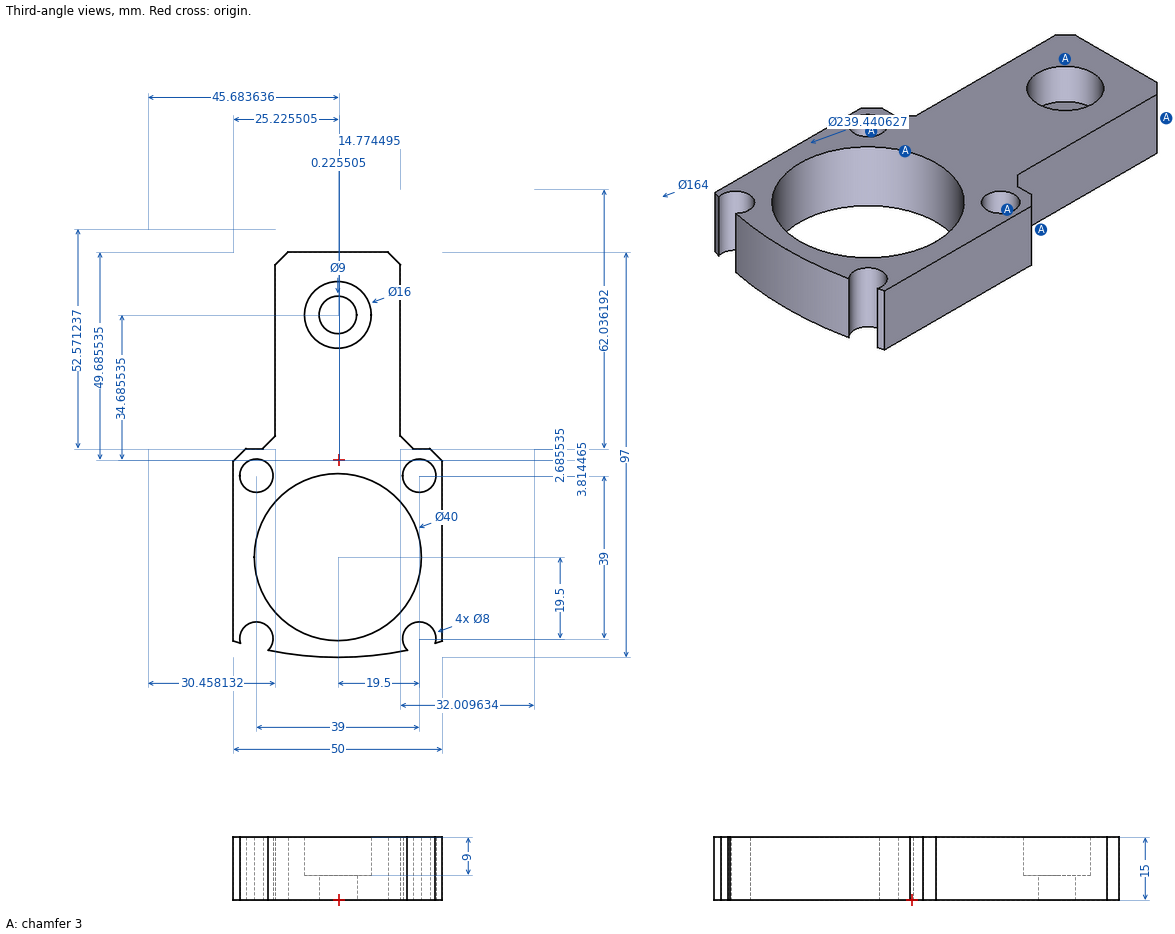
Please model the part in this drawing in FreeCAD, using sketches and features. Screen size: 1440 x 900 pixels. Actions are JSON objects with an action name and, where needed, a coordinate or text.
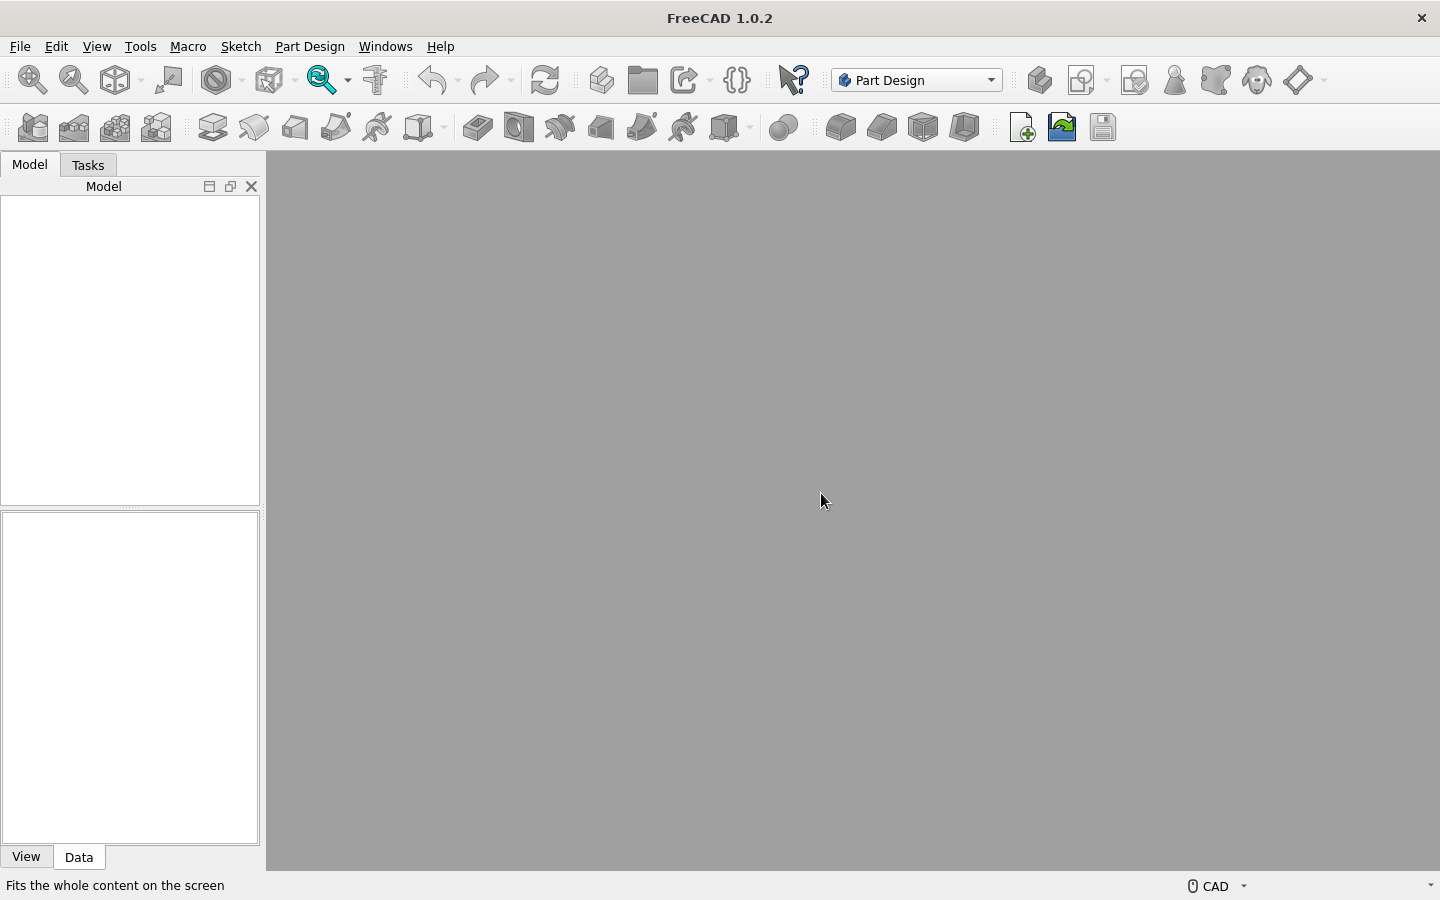
{"action": "left_click", "coordinate": [1021, 128]}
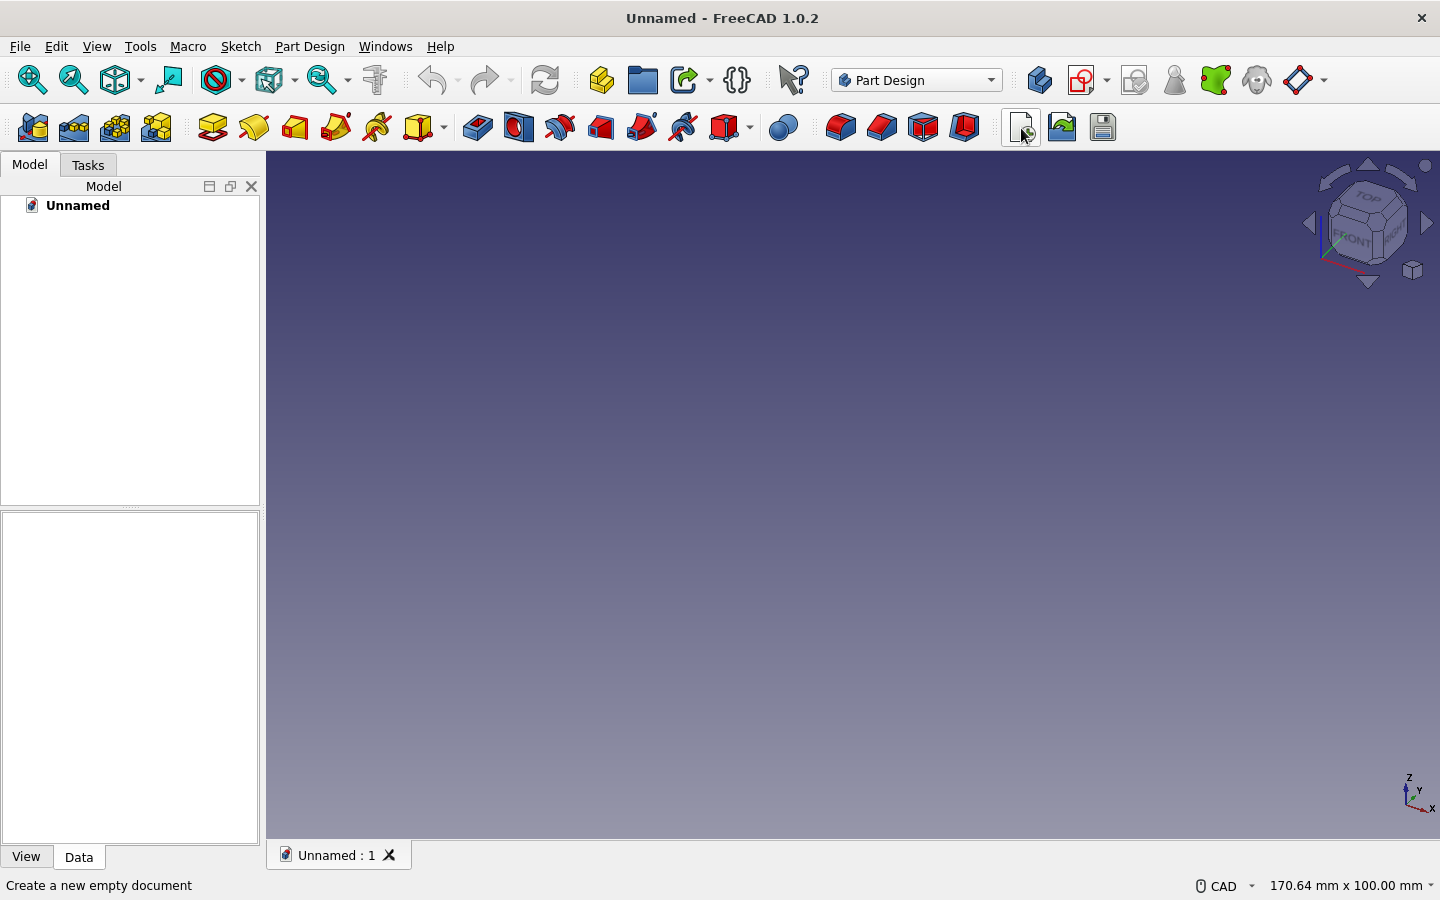
{"action": "left_click", "coordinate": [1080, 80]}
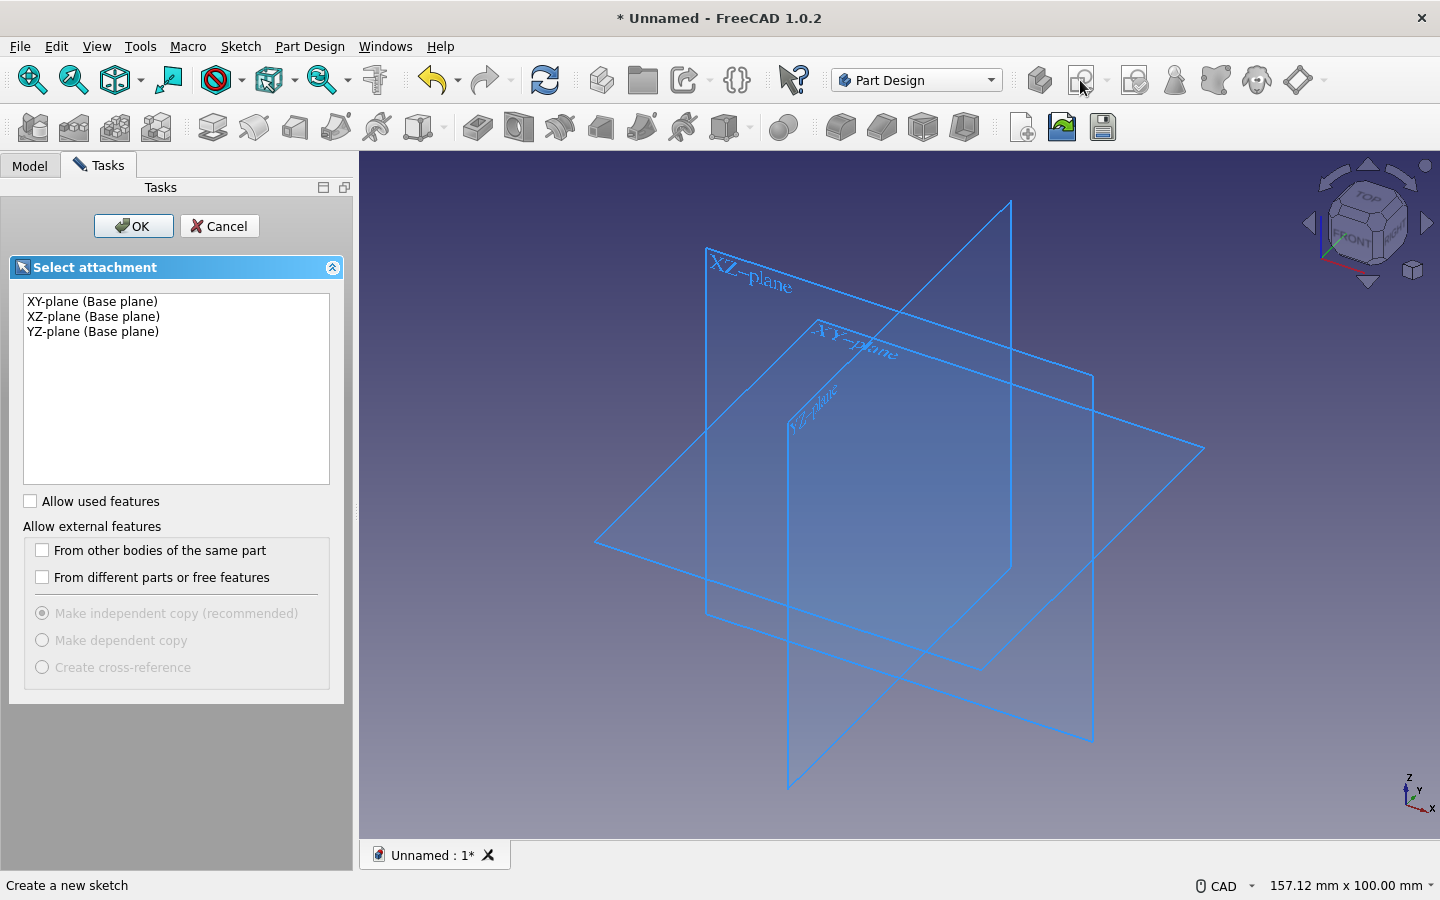
{"action": "left_click", "coordinate": [84, 302]}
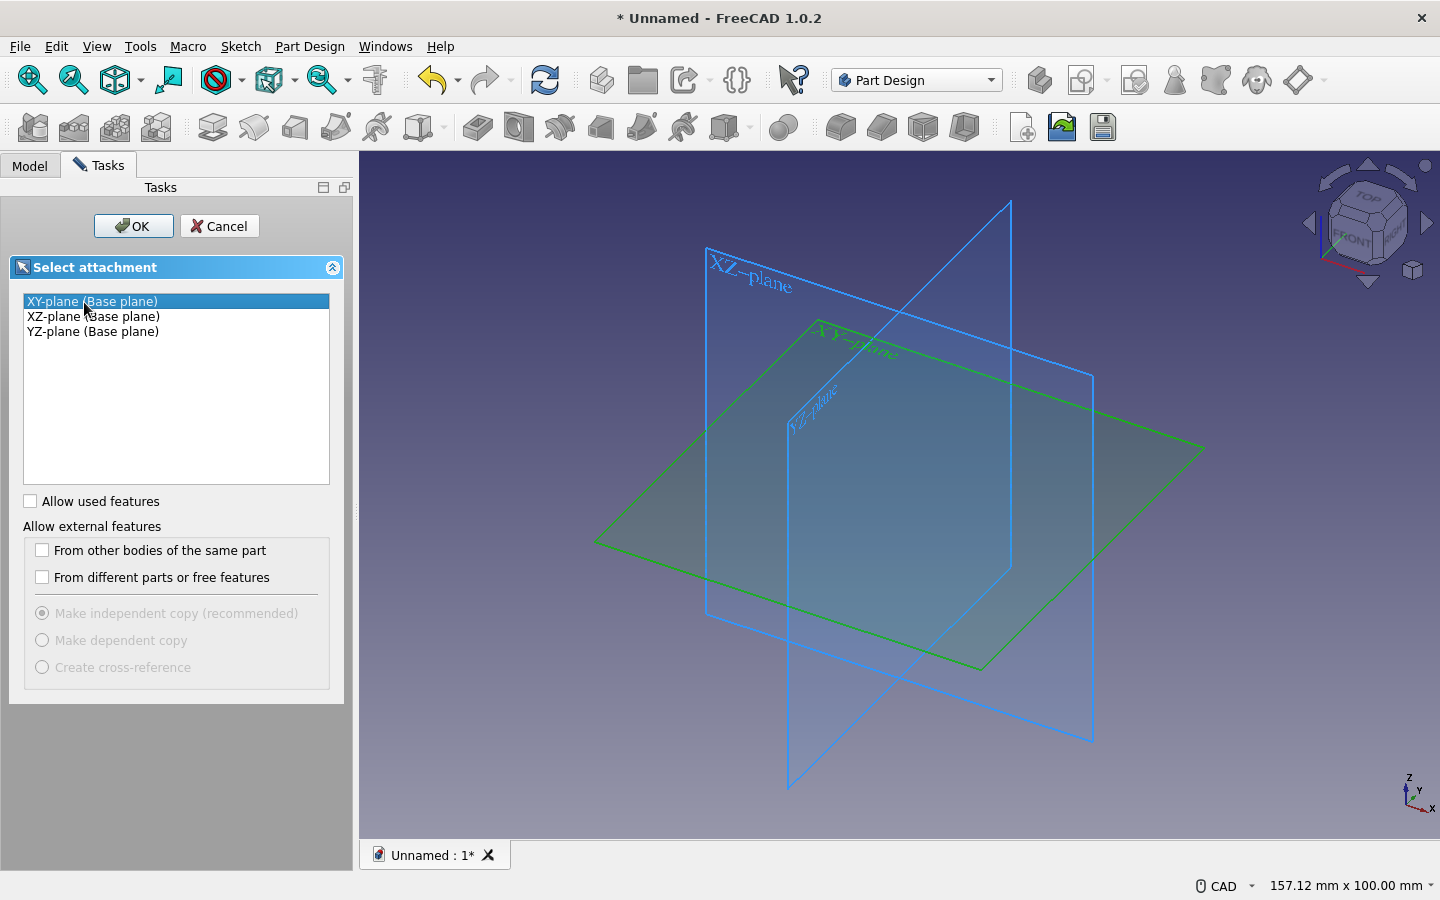
{"action": "left_click", "coordinate": [134, 226]}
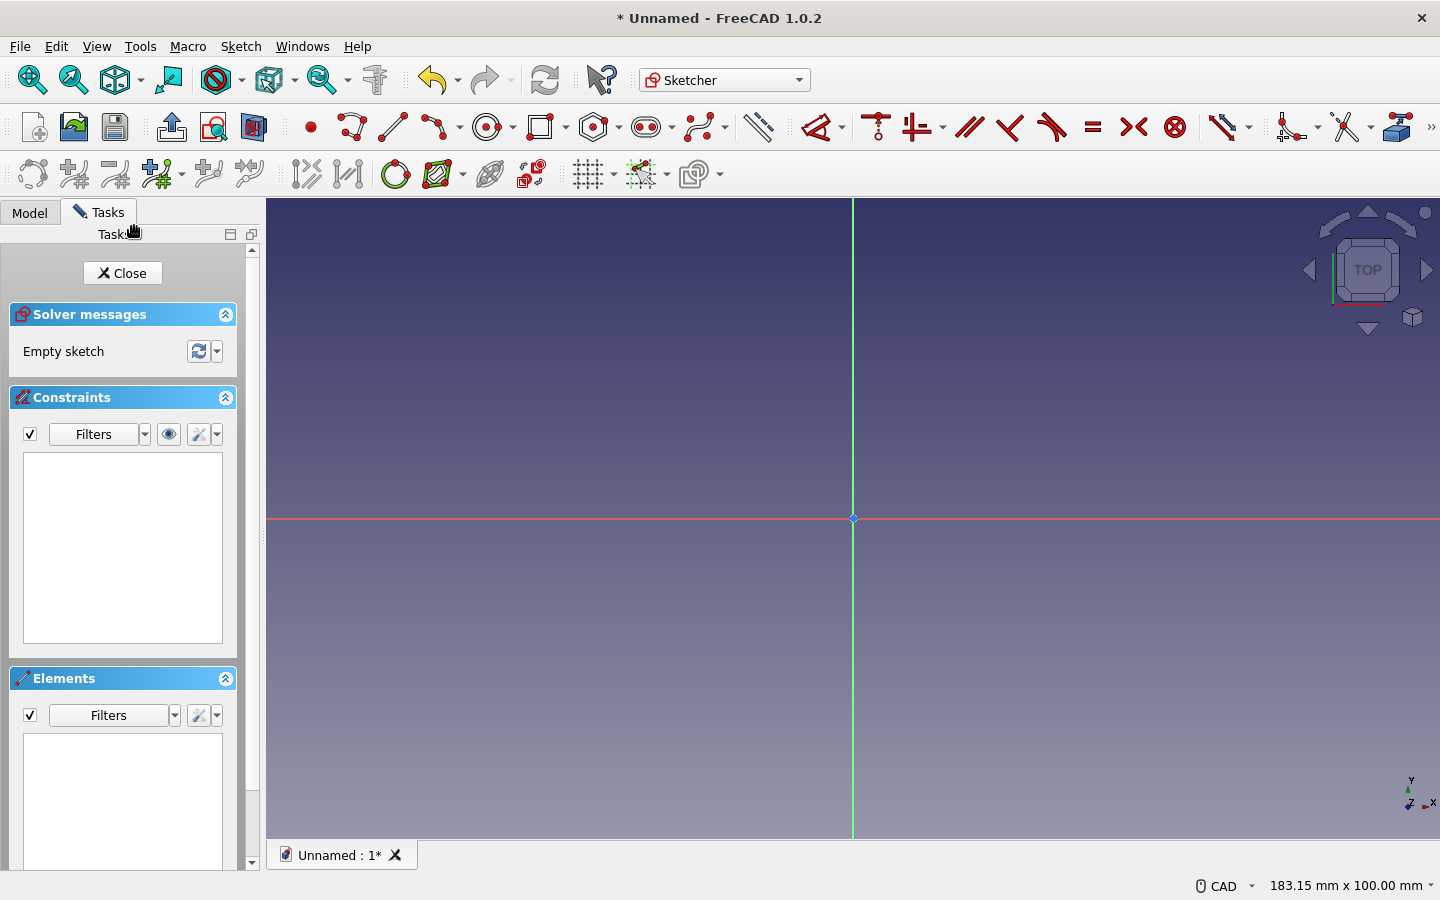
{"action": "scroll", "coordinate": [648, 534], "scroll_direction": "down", "scroll_amount": 2}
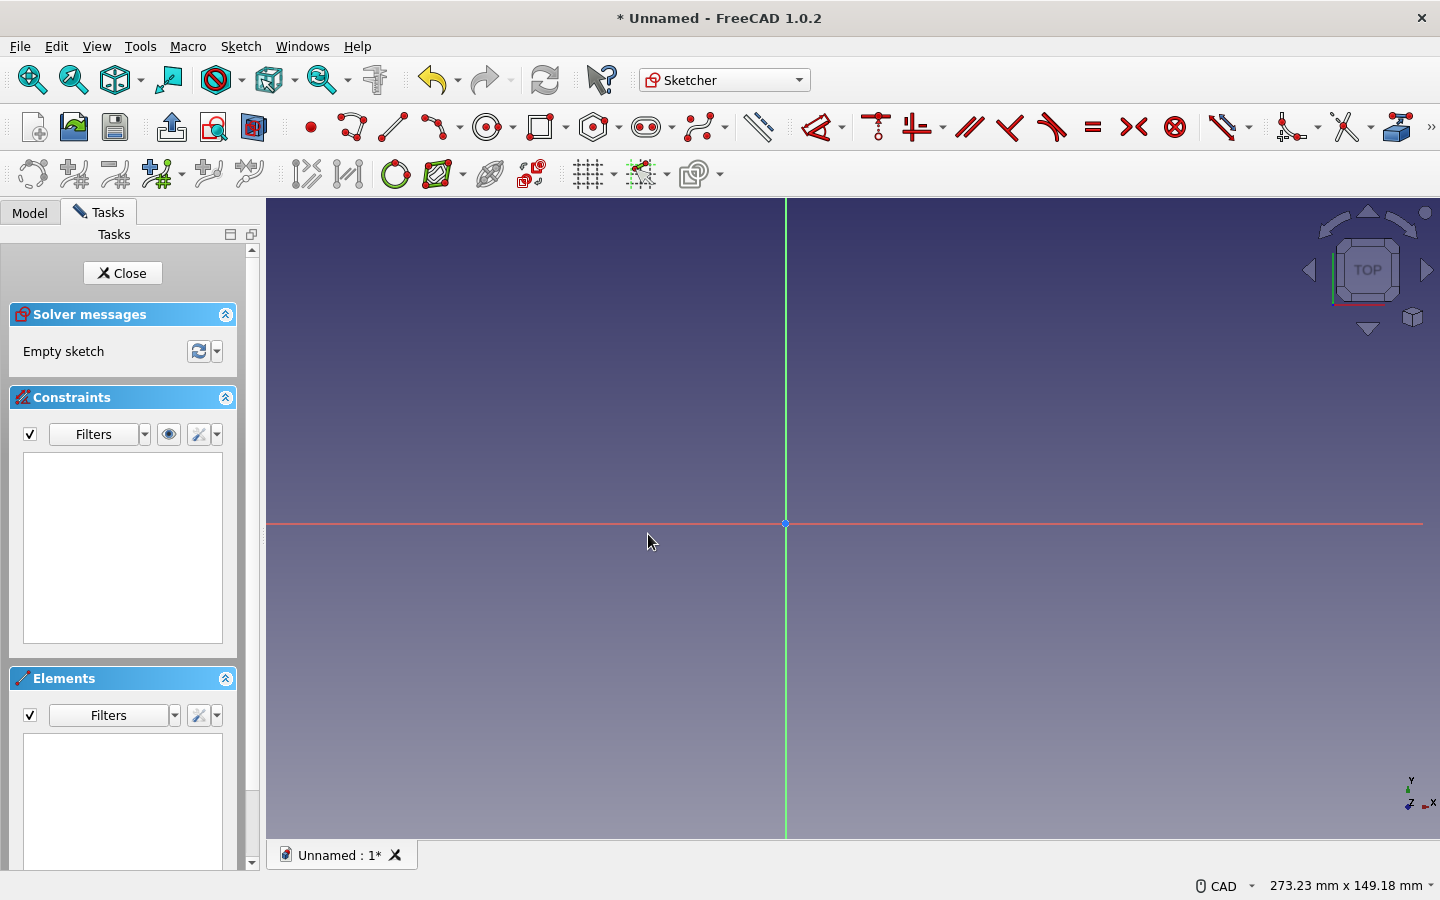
{"action": "key", "text": "g r"}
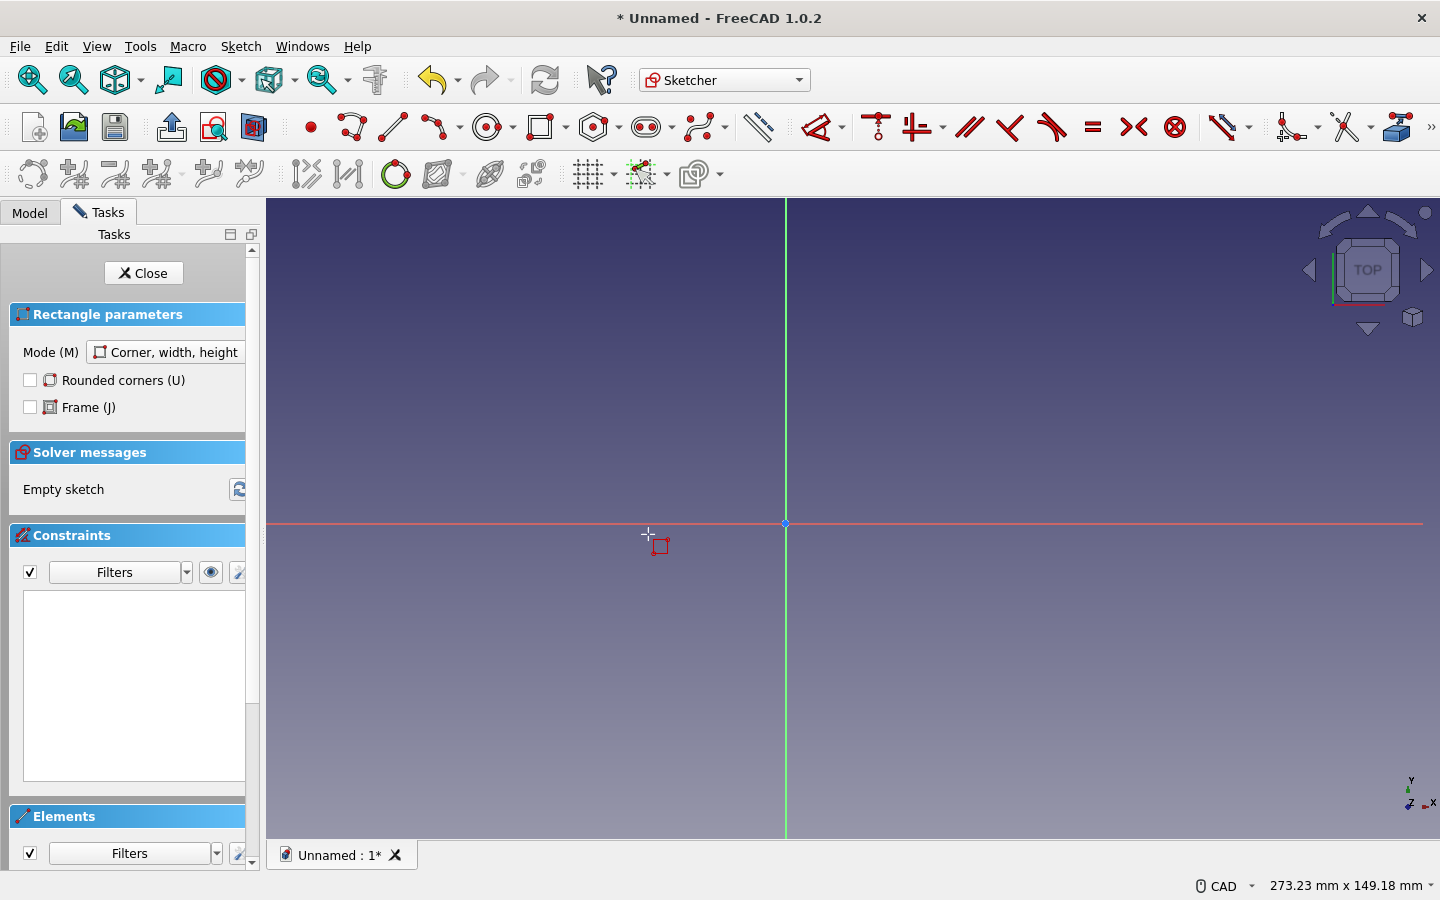
{"action": "left_click", "coordinate": [677, 310]}
{"action": "mouse_move", "coordinate": [892, 727]}